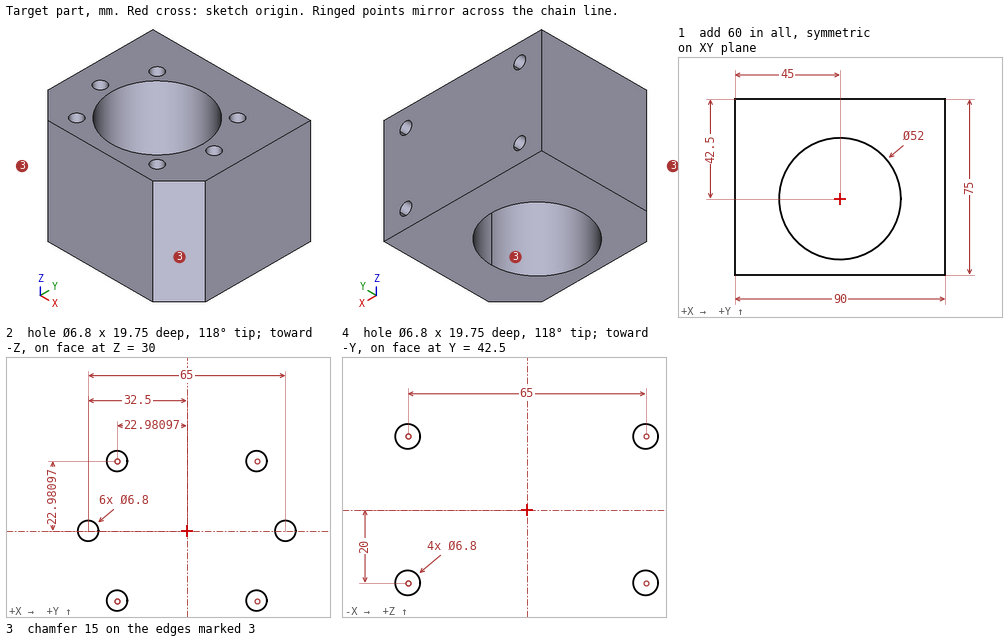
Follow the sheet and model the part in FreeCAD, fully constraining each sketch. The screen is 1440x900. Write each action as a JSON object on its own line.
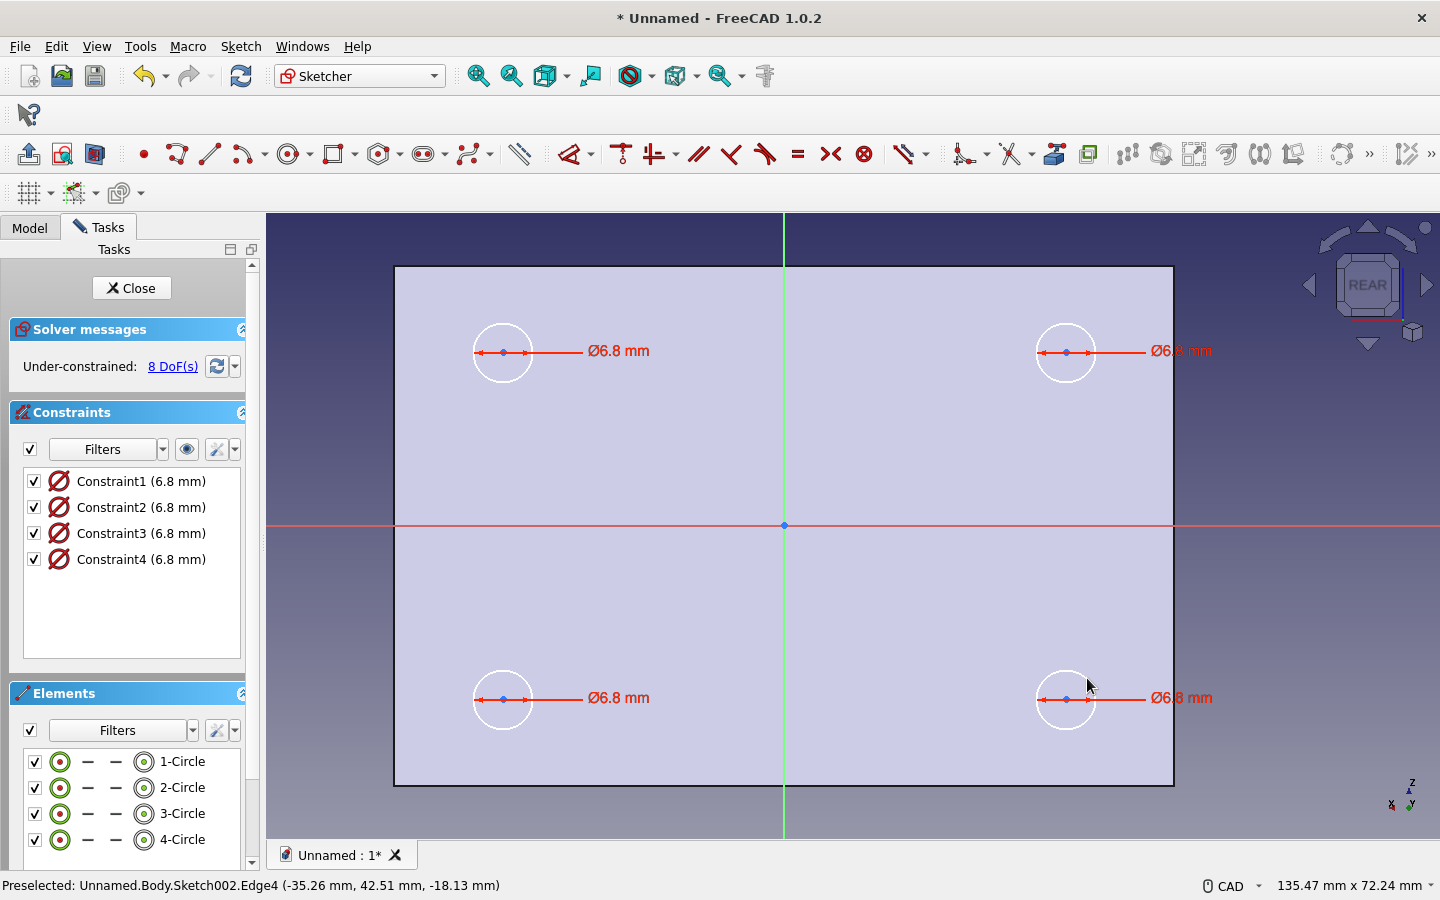
{"action": "left_click", "coordinate": [503, 700]}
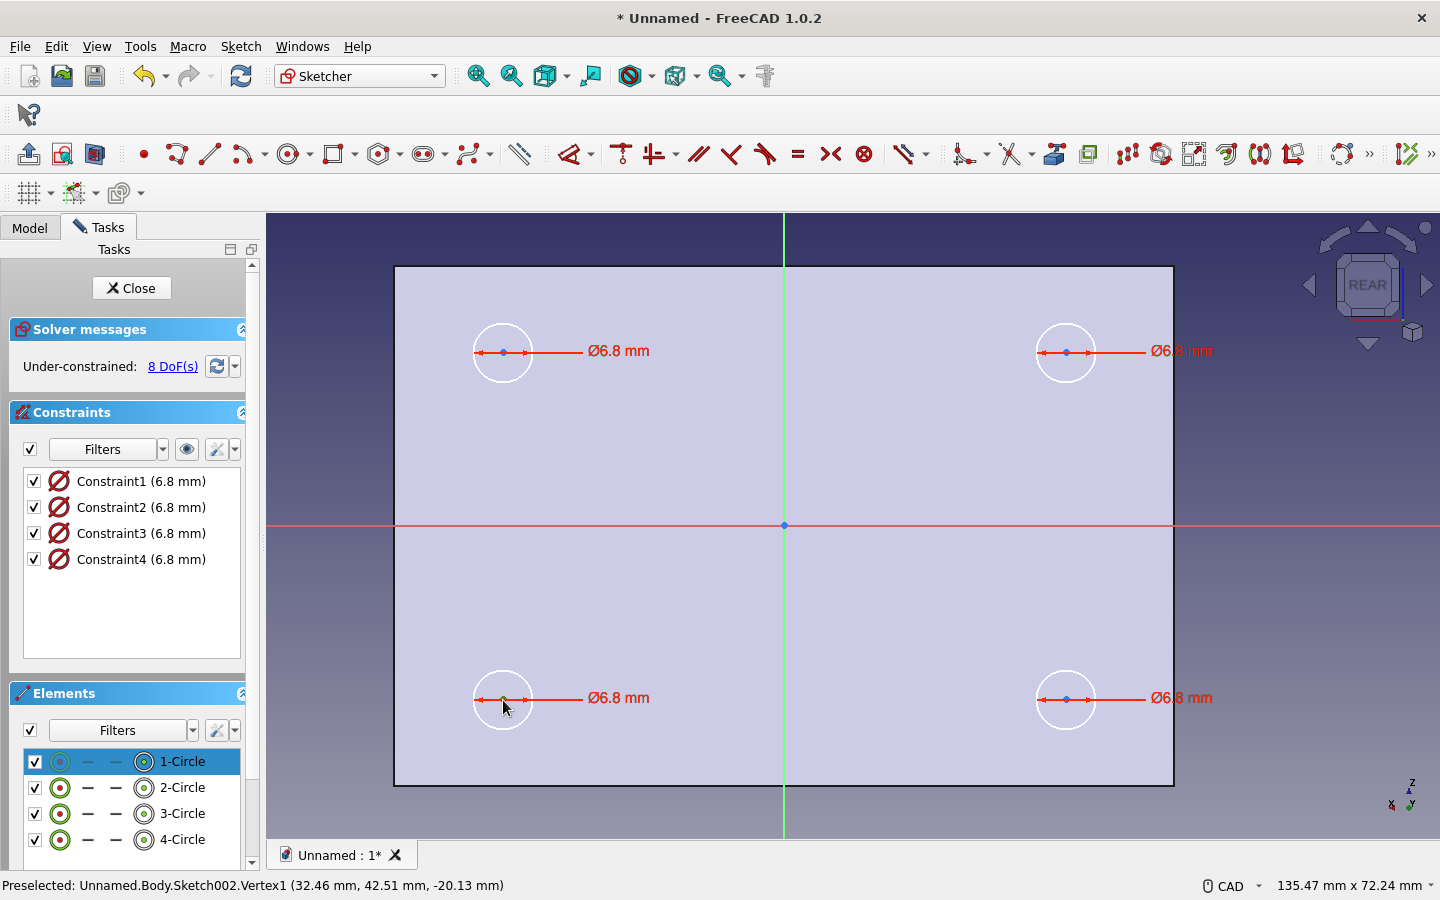
{"action": "left_click", "coordinate": [503, 353]}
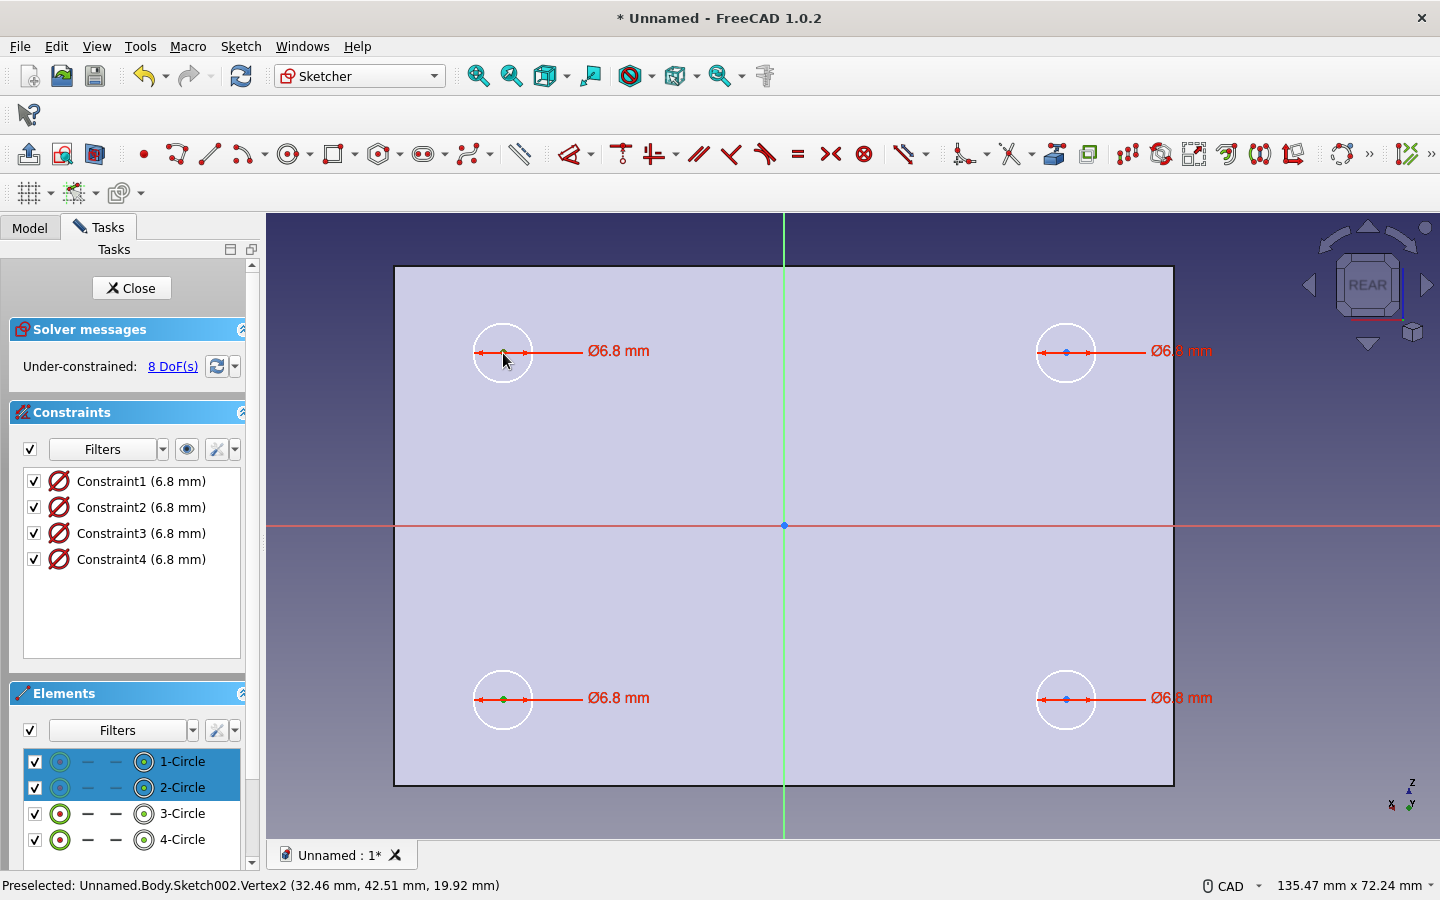
{"action": "left_click", "coordinate": [364, 526]}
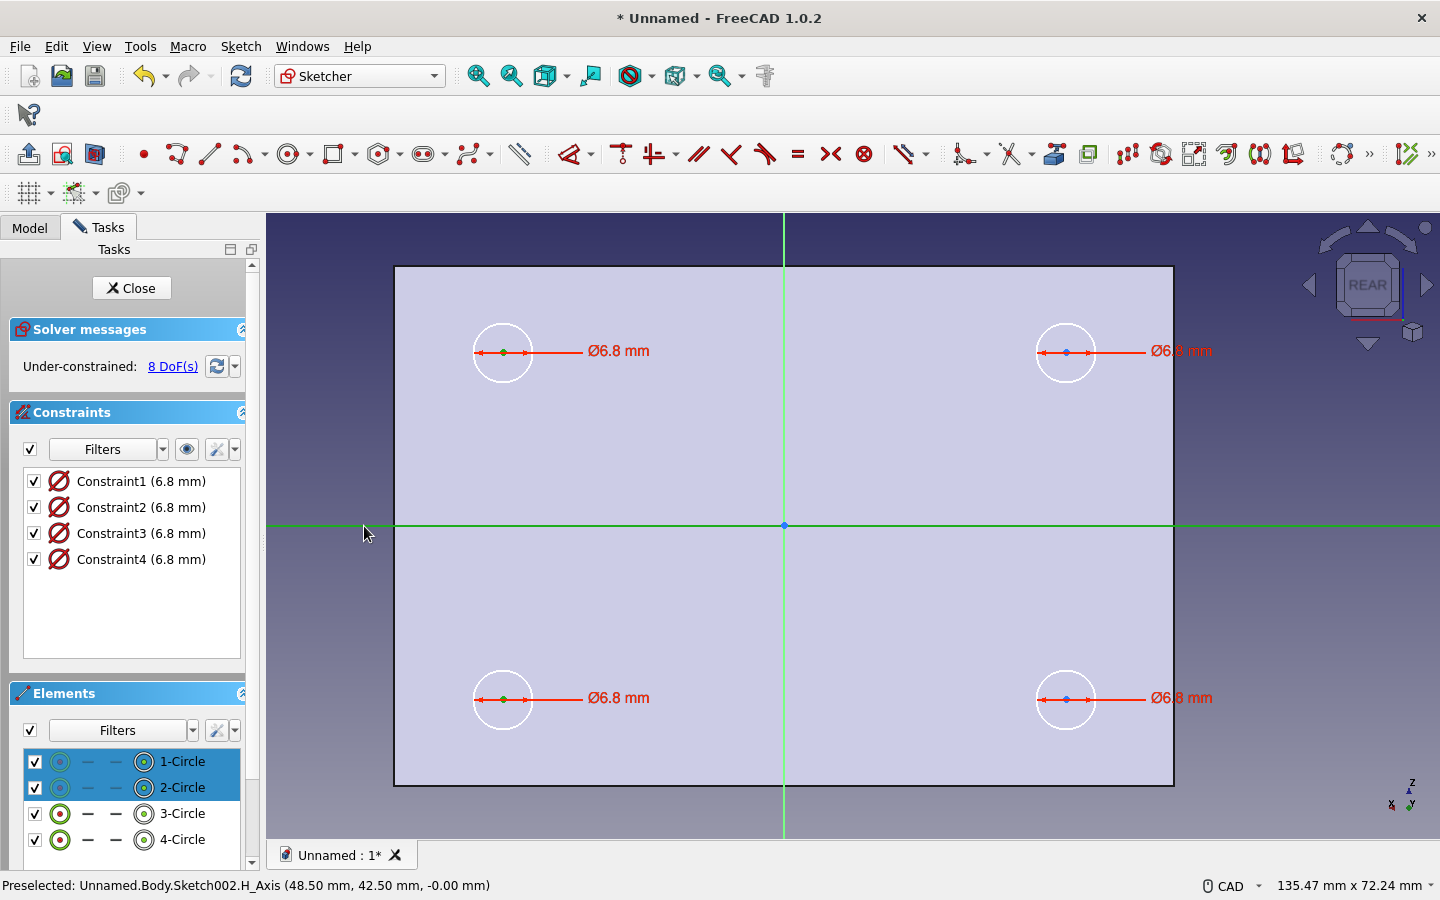
{"action": "left_click", "coordinate": [831, 154]}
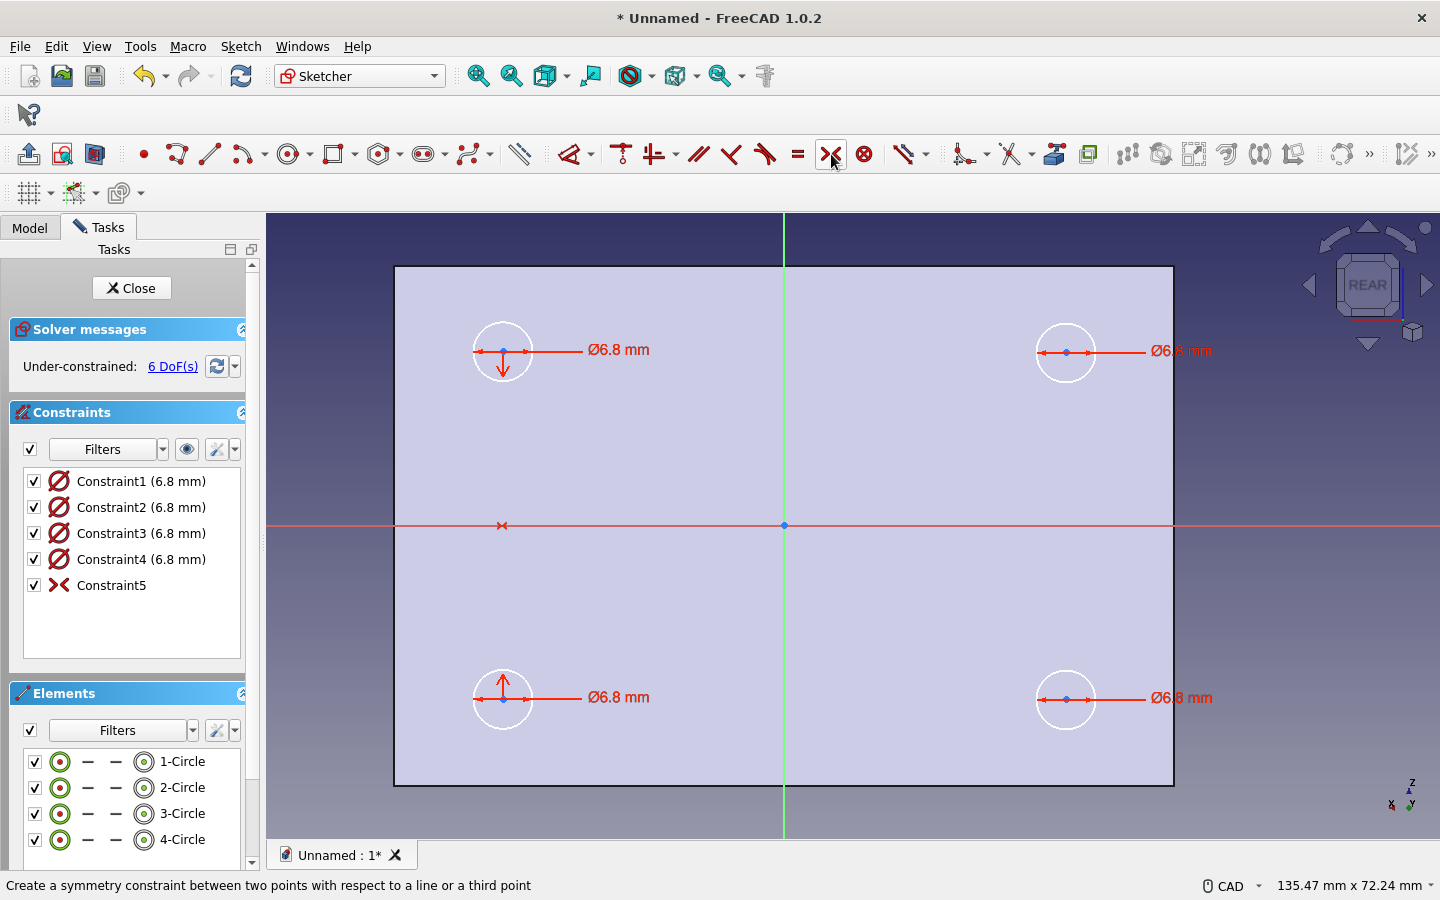
{"action": "left_click", "coordinate": [503, 352]}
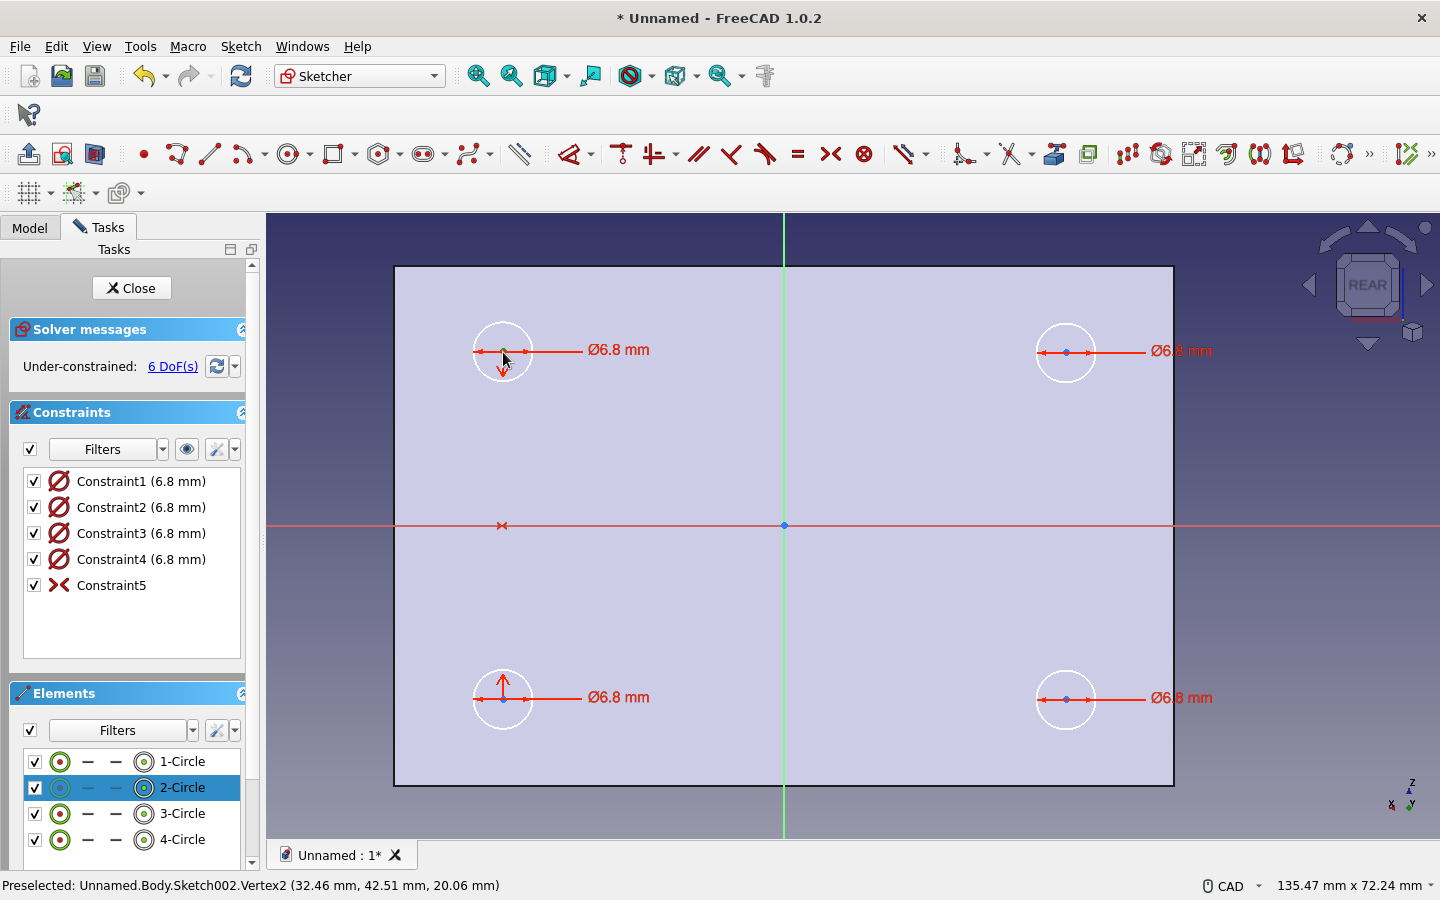
{"action": "left_click", "coordinate": [1066, 353]}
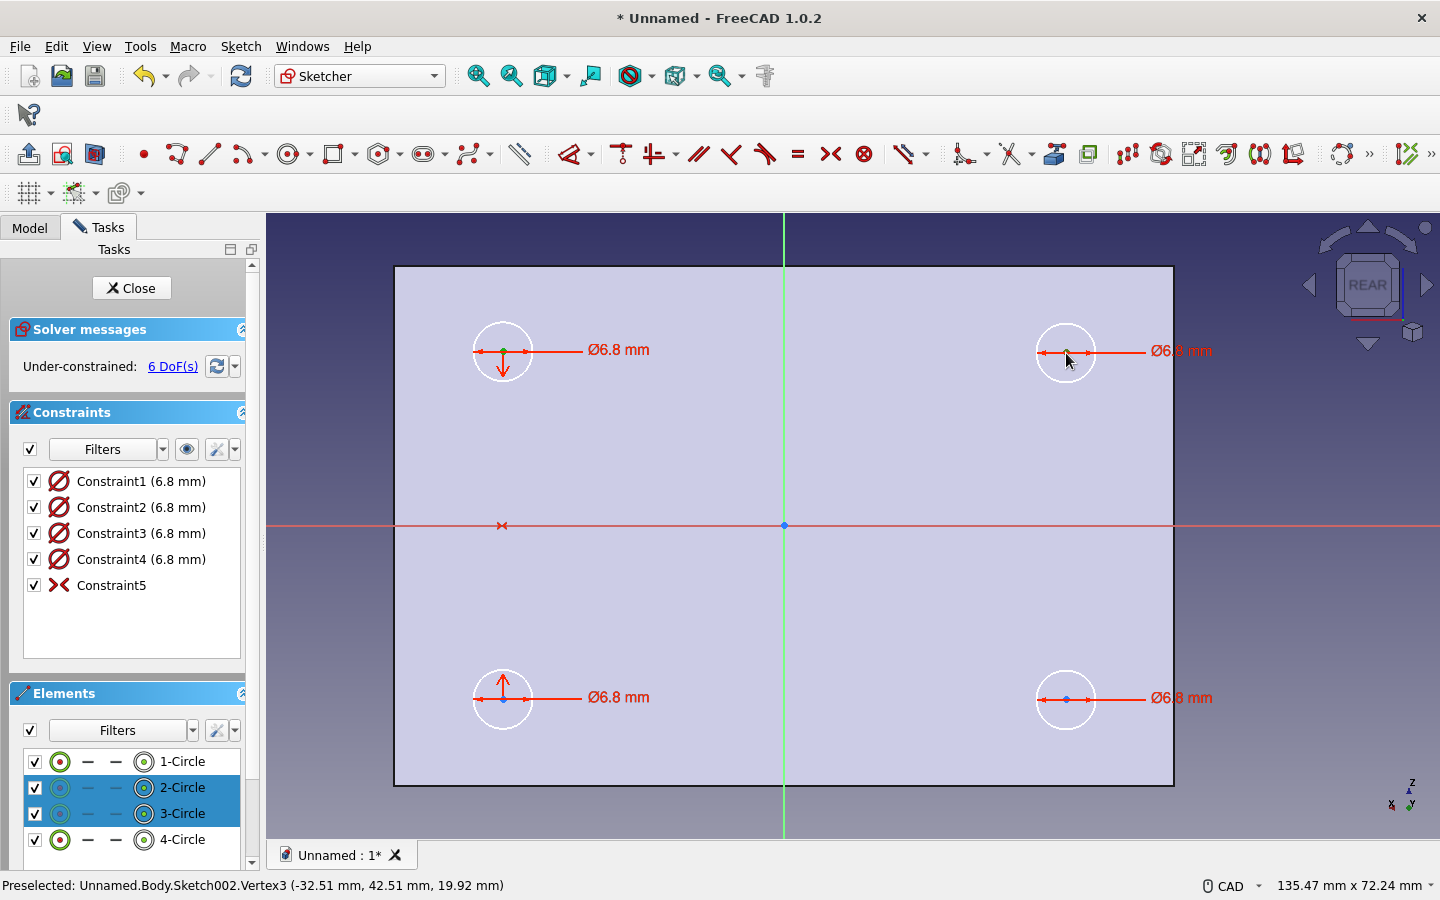
{"action": "left_click", "coordinate": [784, 770]}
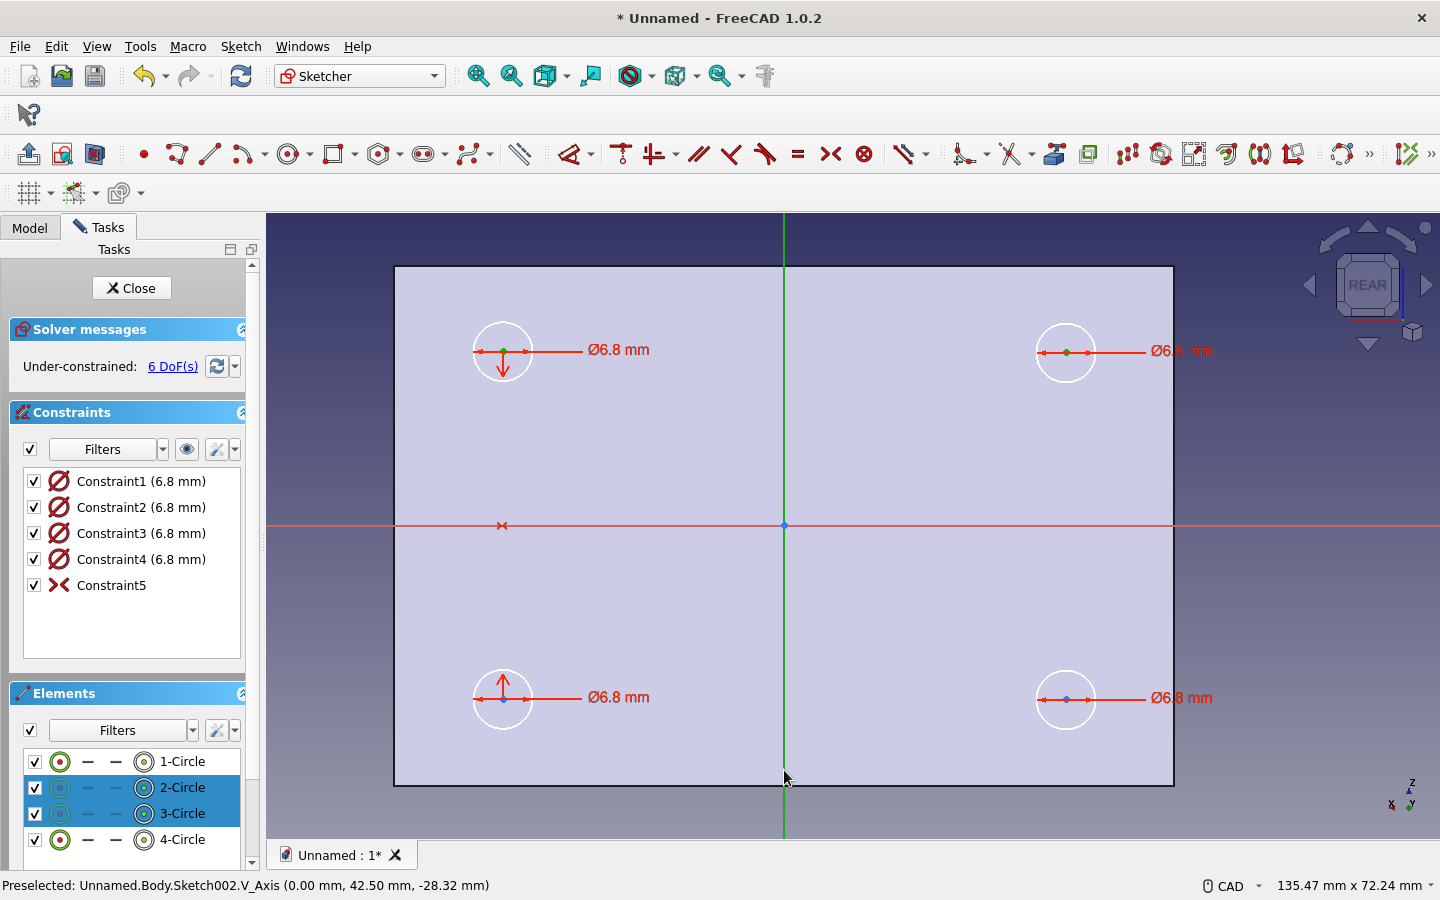
{"action": "left_click", "coordinate": [831, 154]}